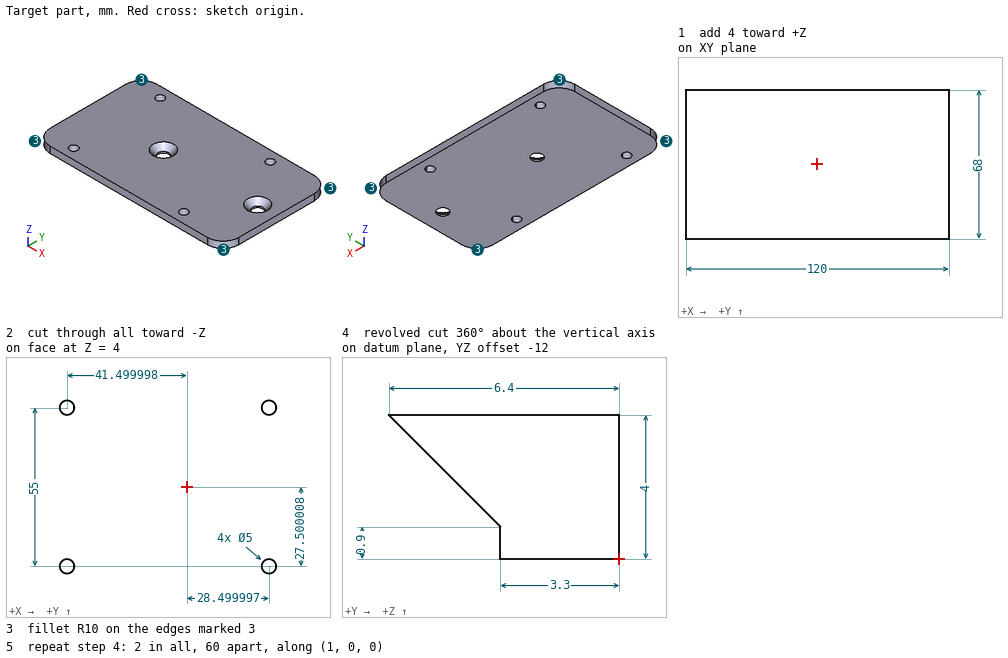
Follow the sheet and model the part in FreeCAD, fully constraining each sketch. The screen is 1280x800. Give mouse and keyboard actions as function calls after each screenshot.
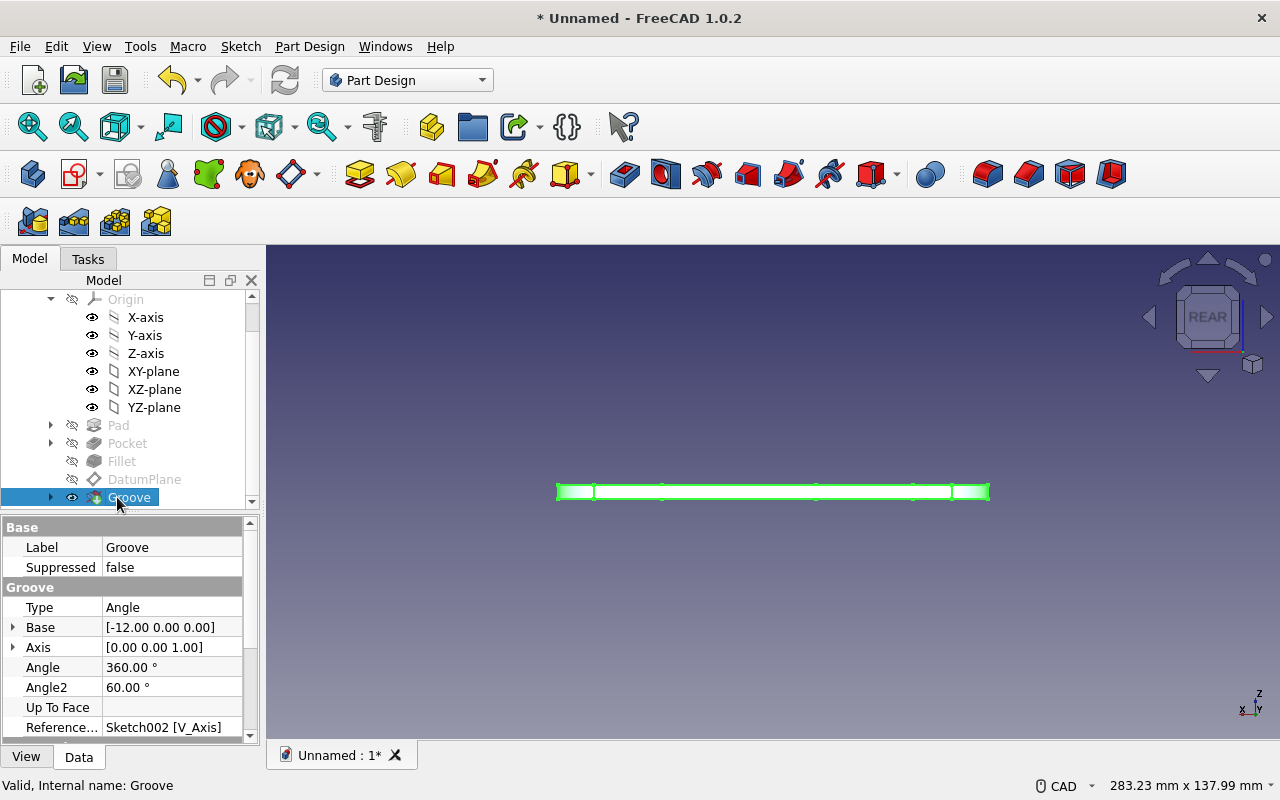
click(74, 222)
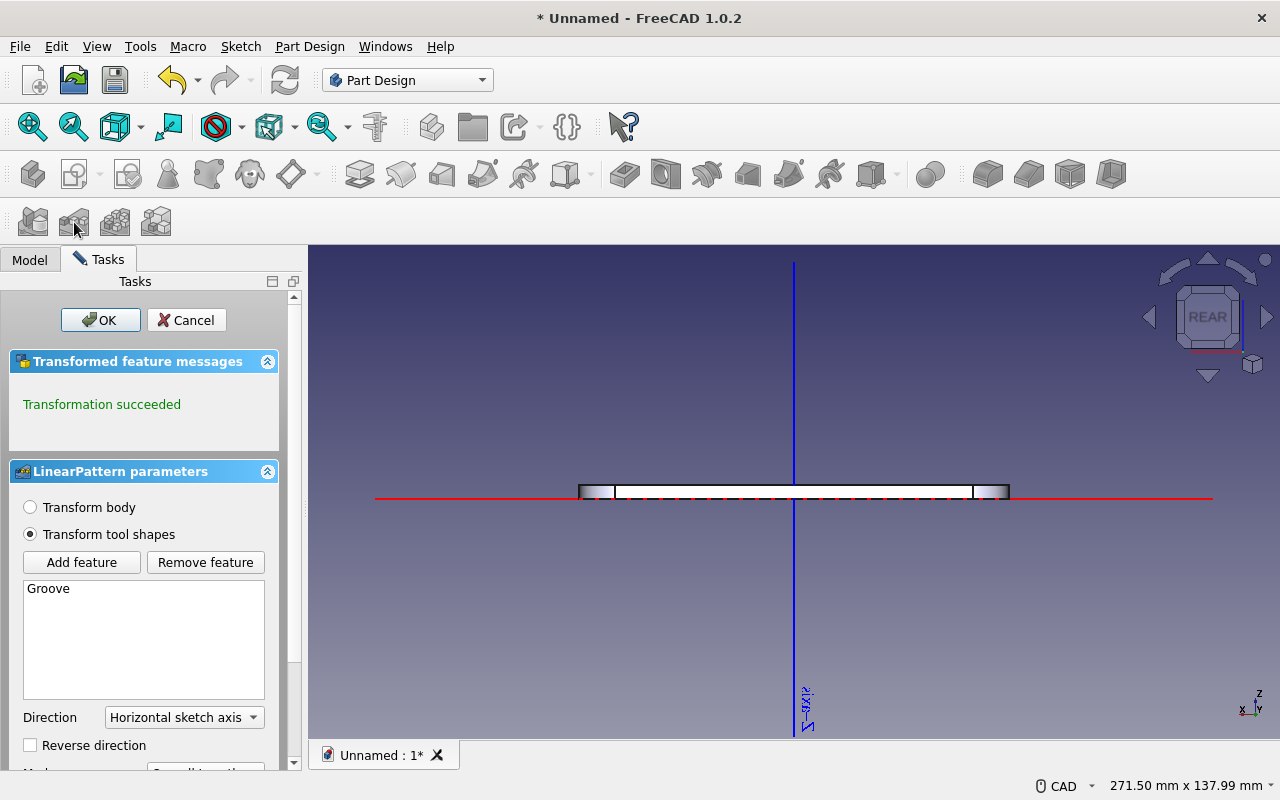
click(185, 718)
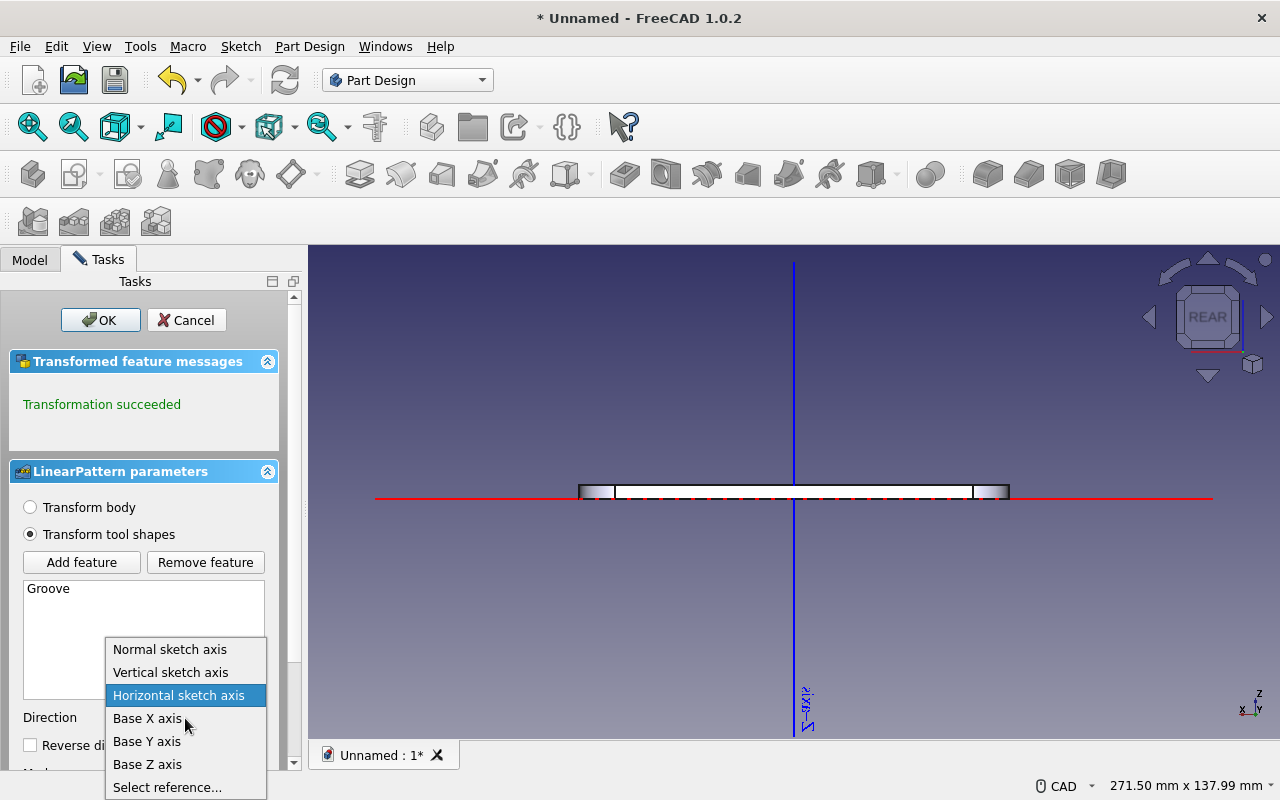
click(184, 718)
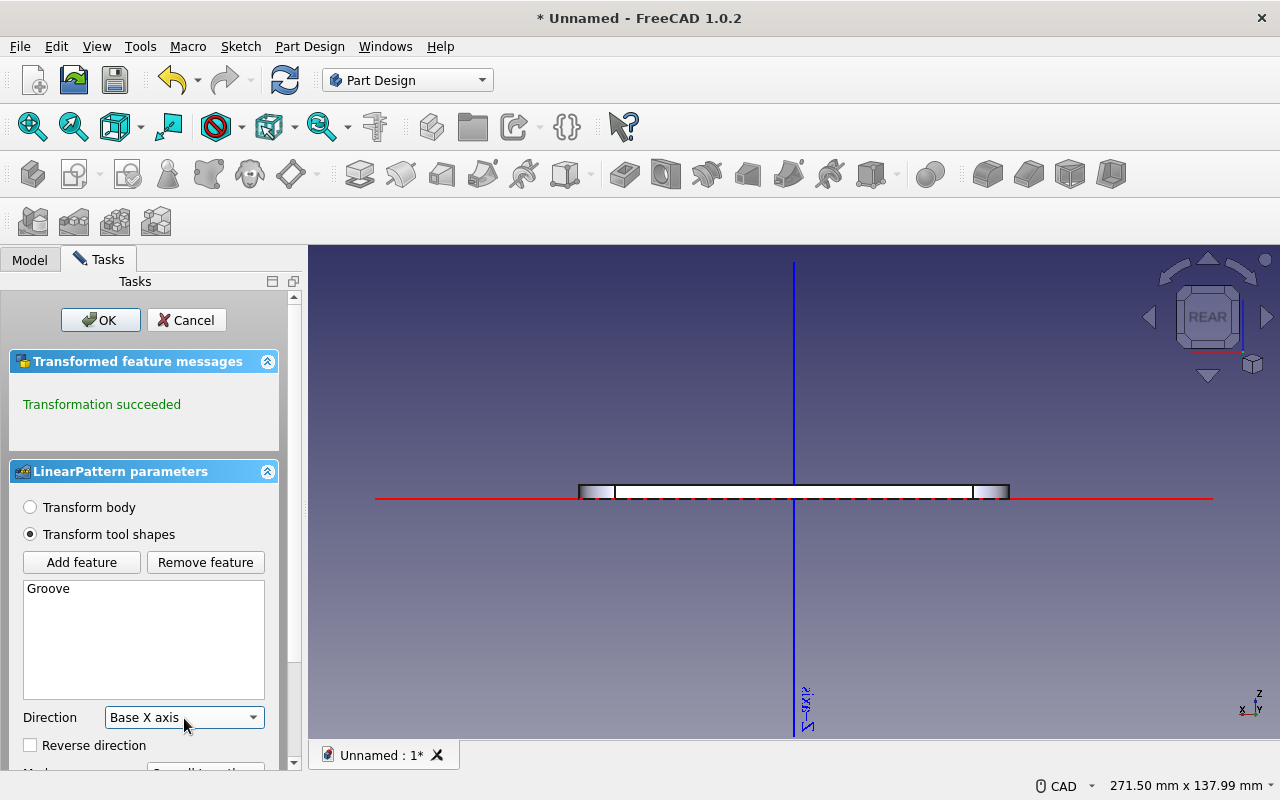
scroll(294, 530, down, 2)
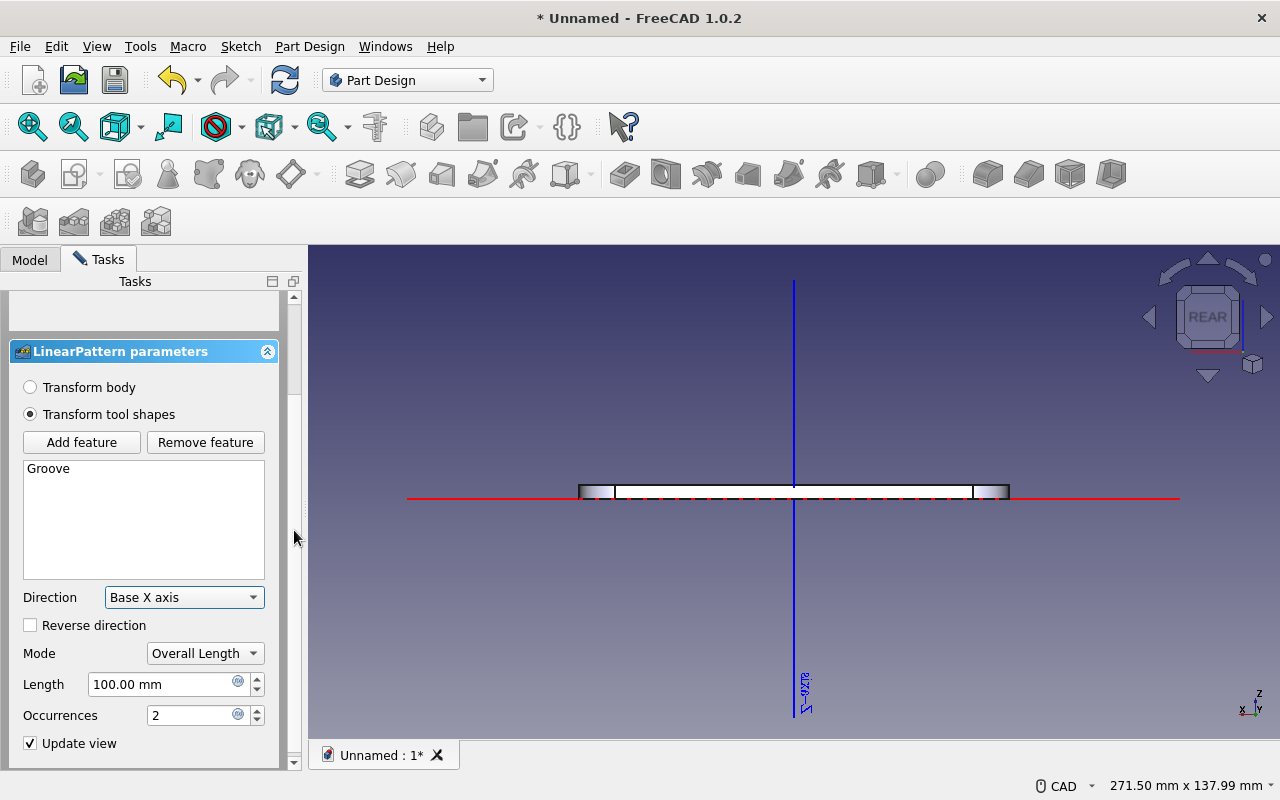
click(206, 654)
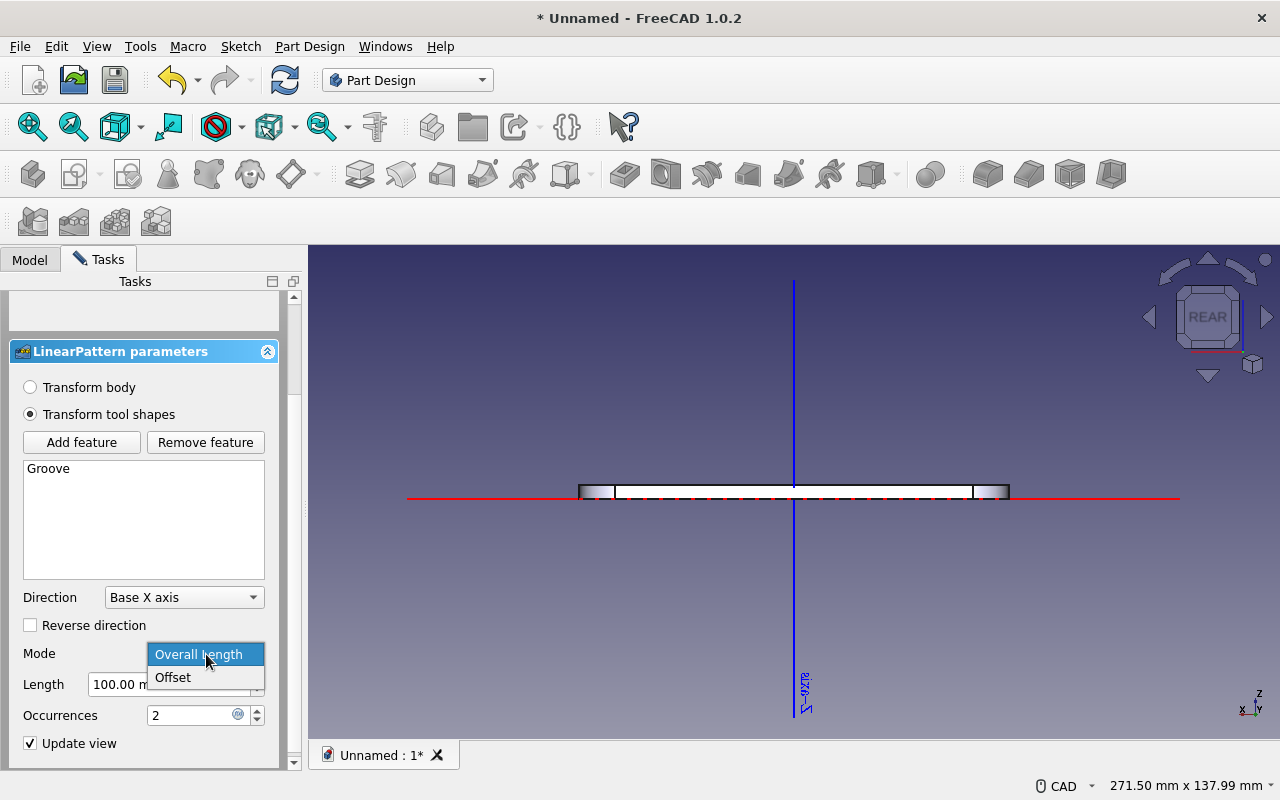
click(204, 678)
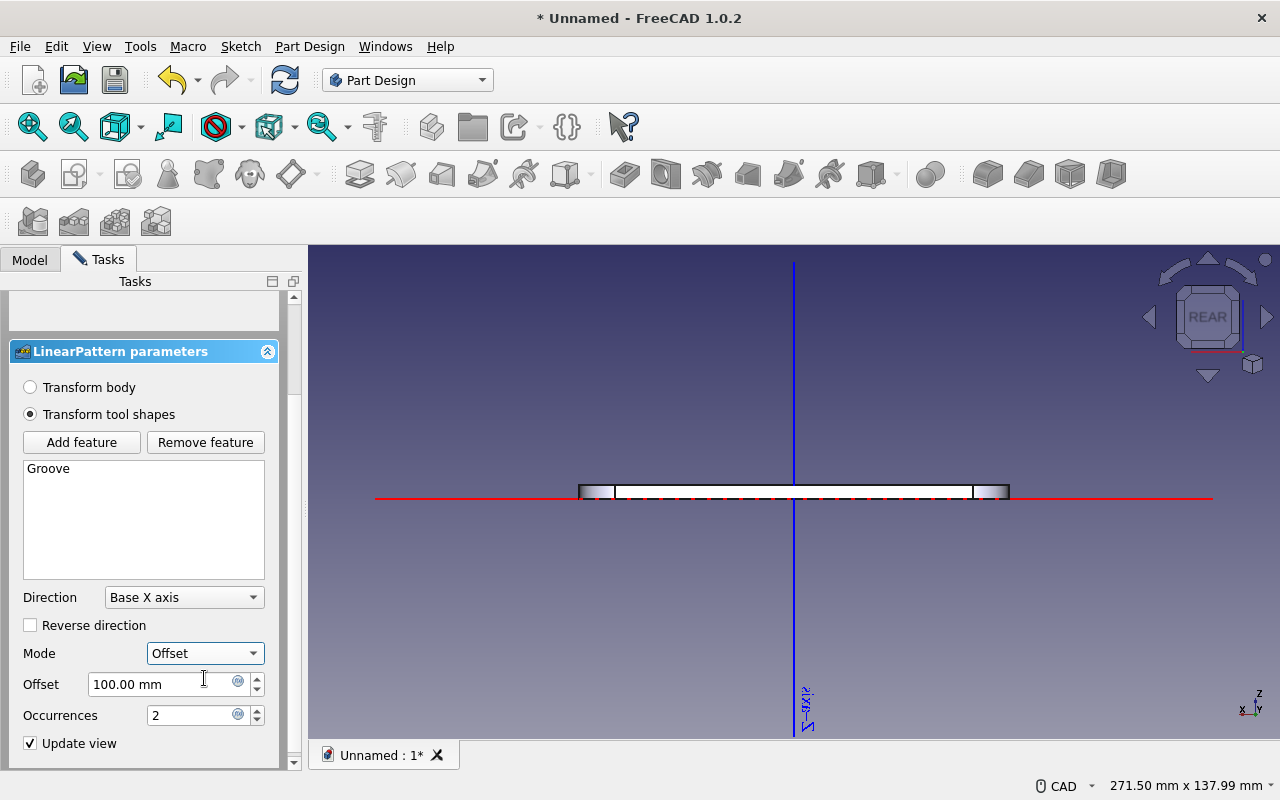
triple_click(170, 684)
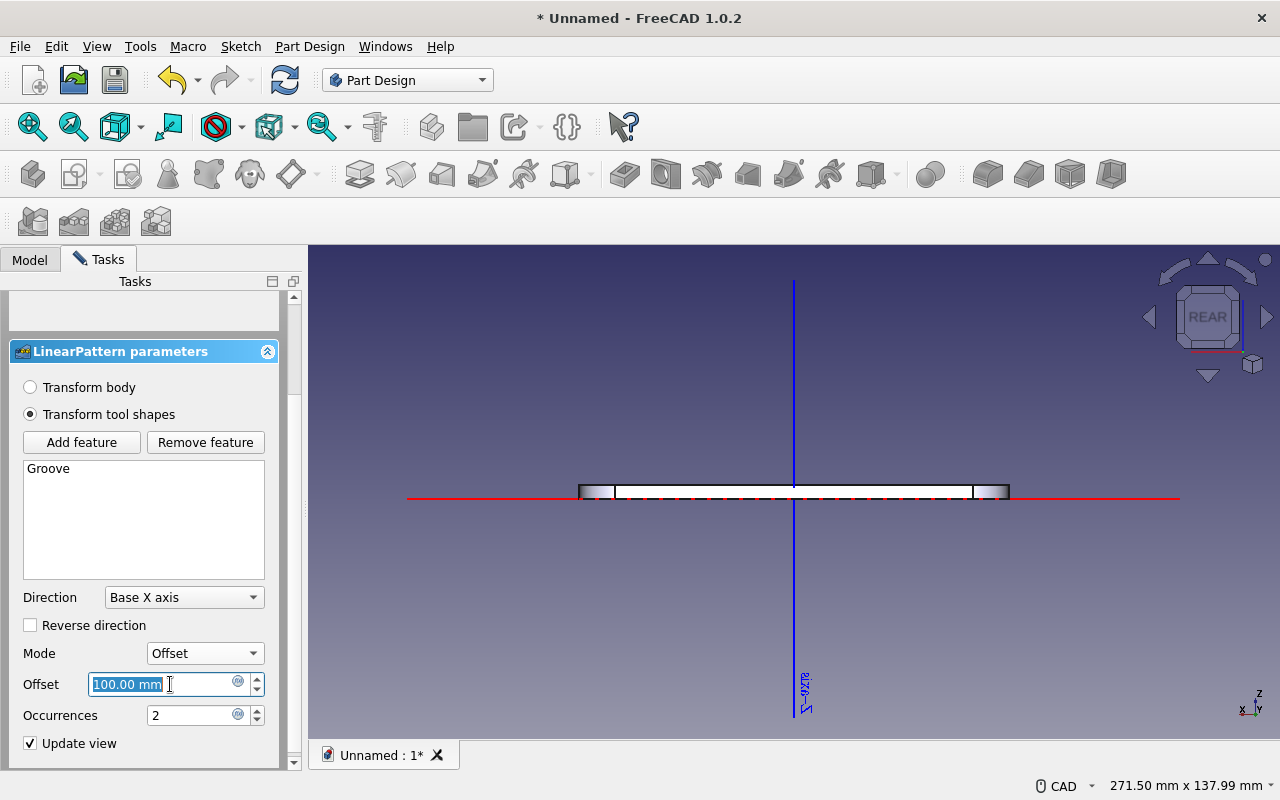
text(60)
key(Tab)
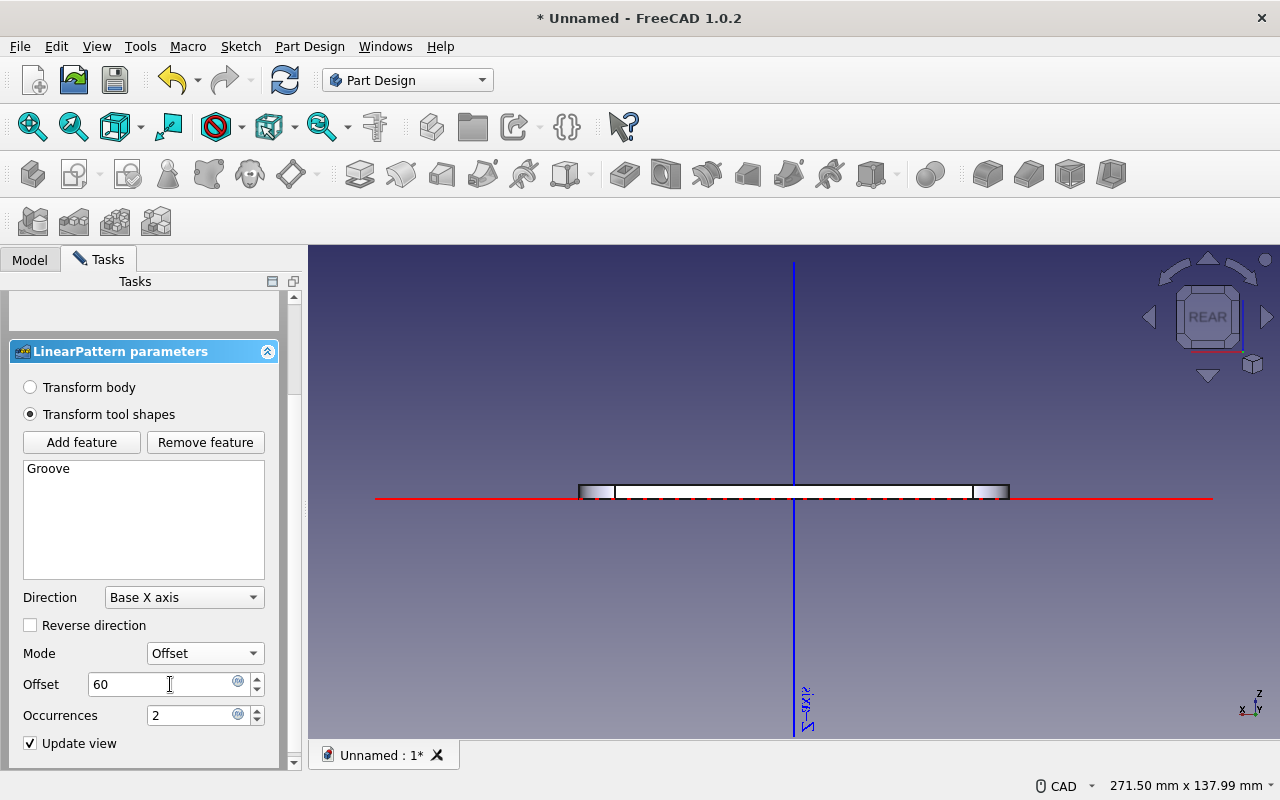
triple_click(199, 716)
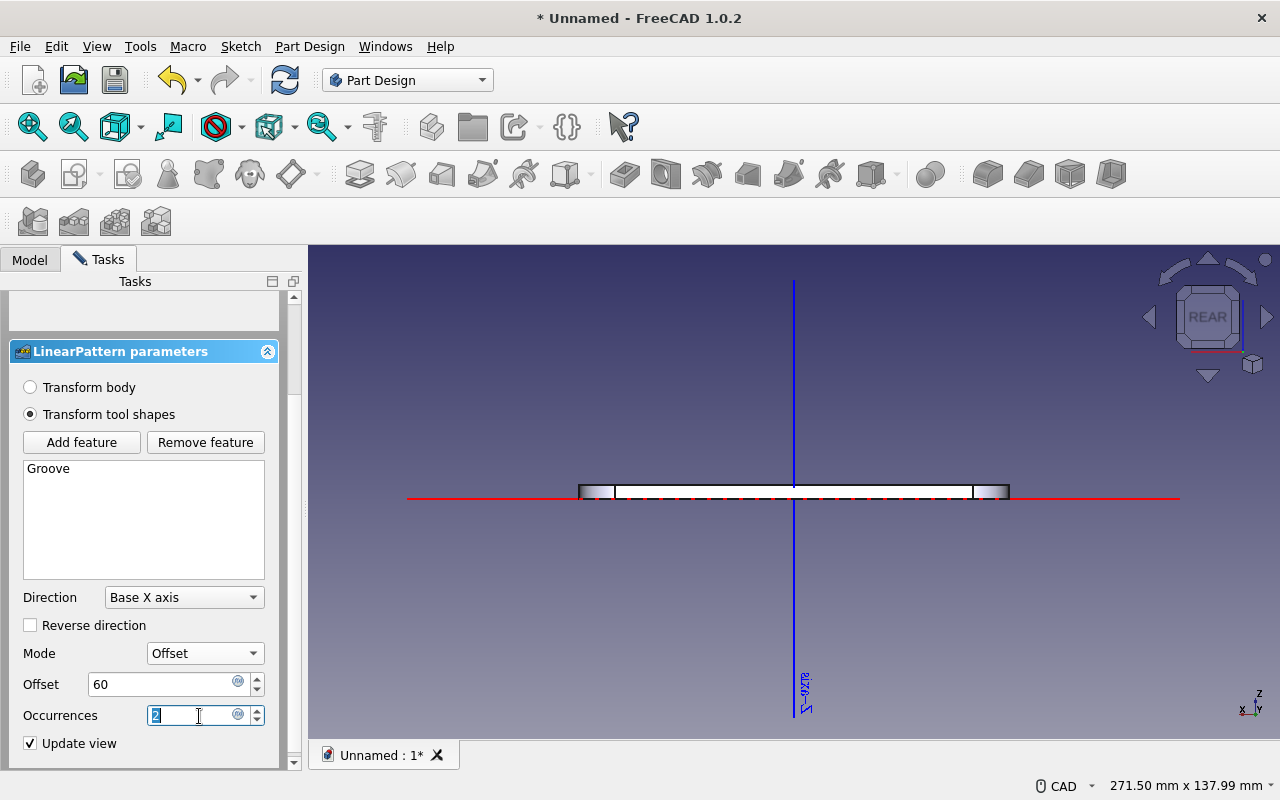
text(2)
key(Tab)